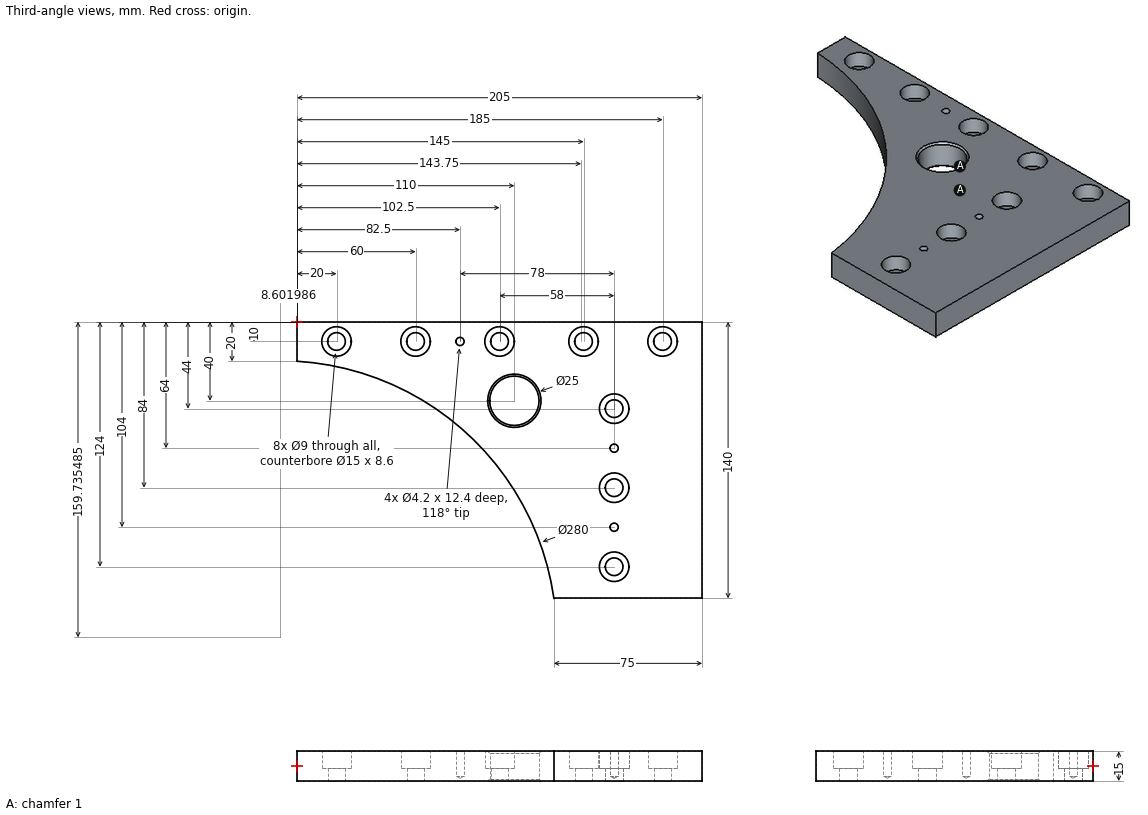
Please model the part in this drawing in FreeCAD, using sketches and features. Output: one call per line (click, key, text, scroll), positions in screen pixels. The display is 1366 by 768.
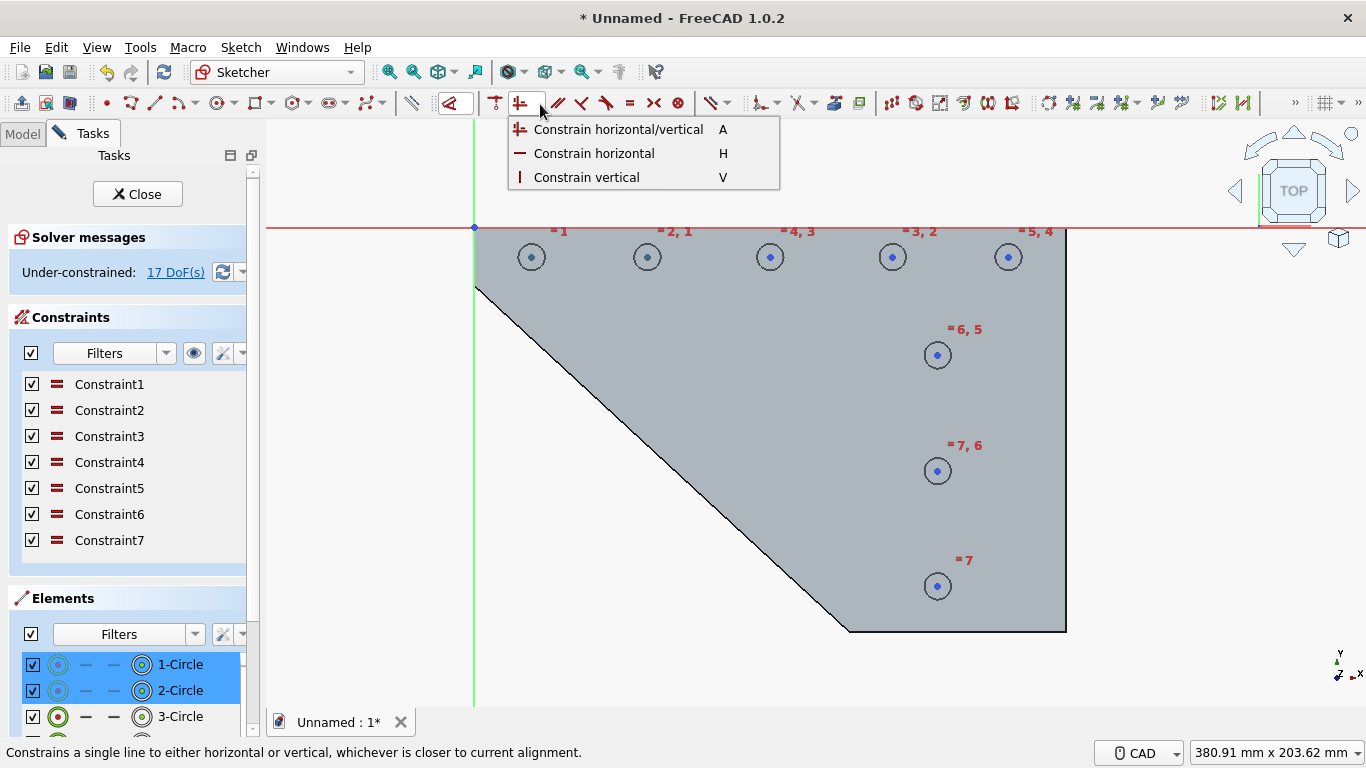
click(644, 153)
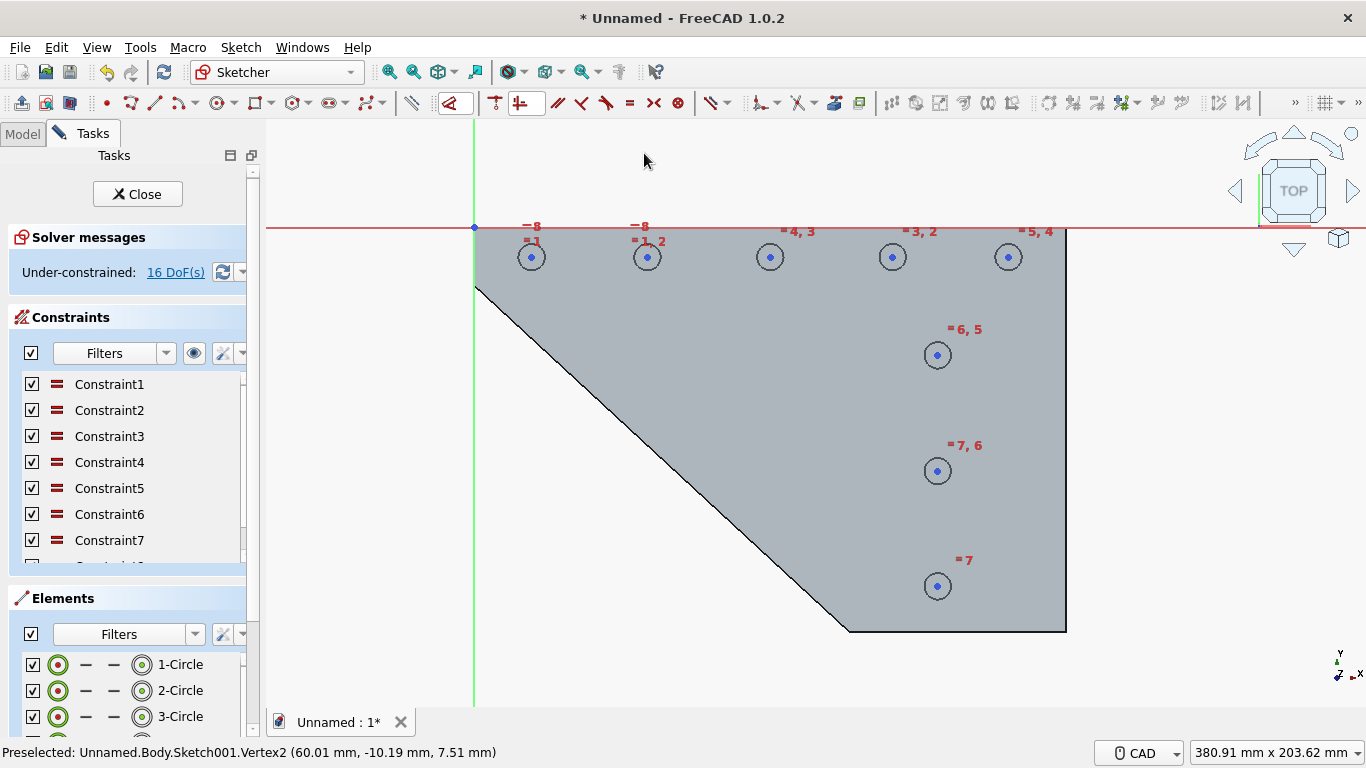
click(647, 257)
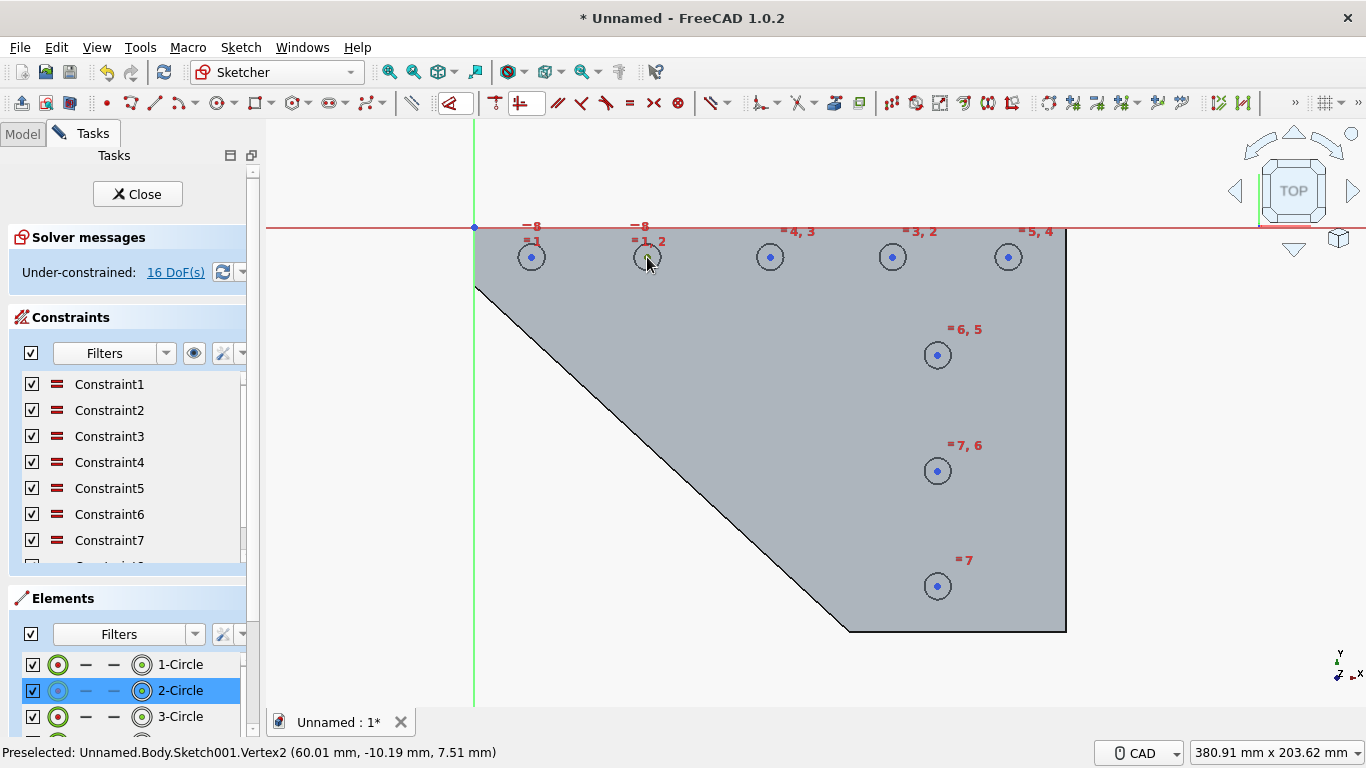
click(893, 257)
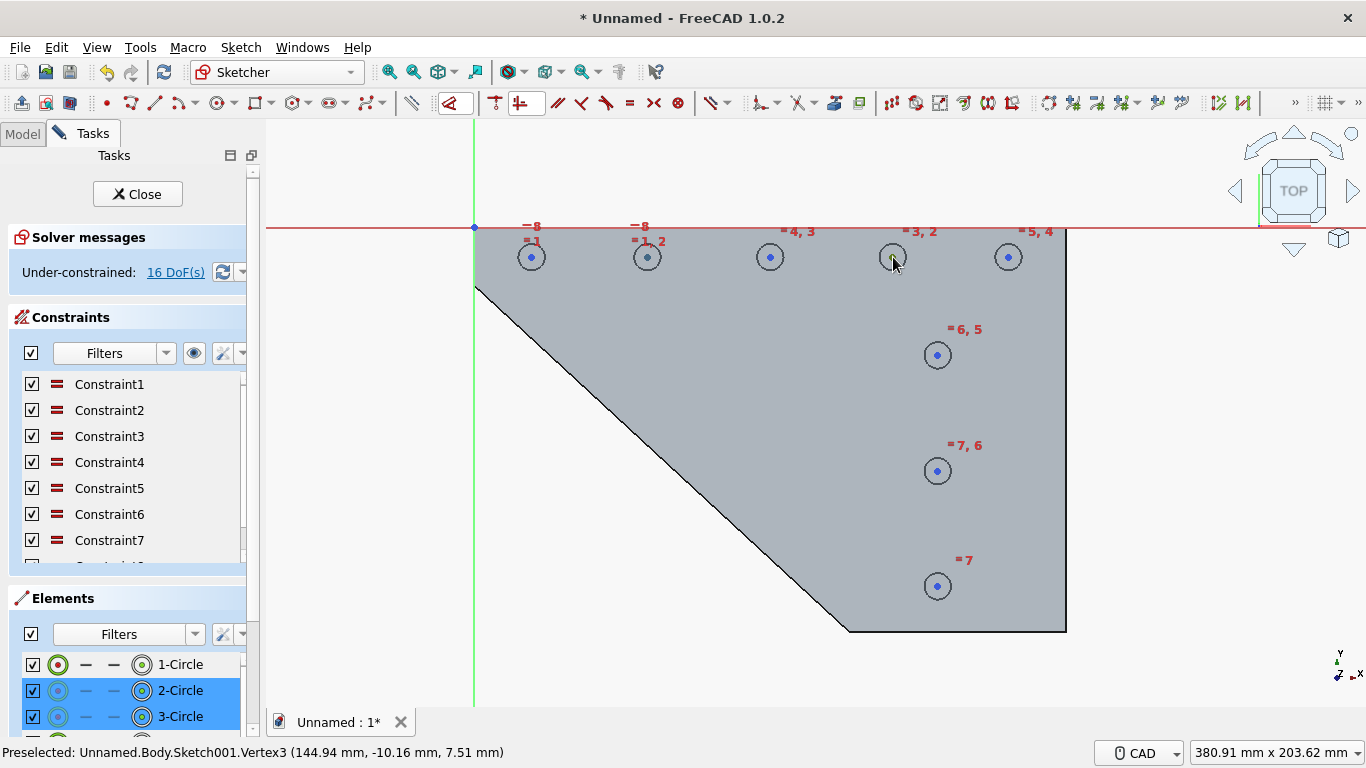
click(540, 104)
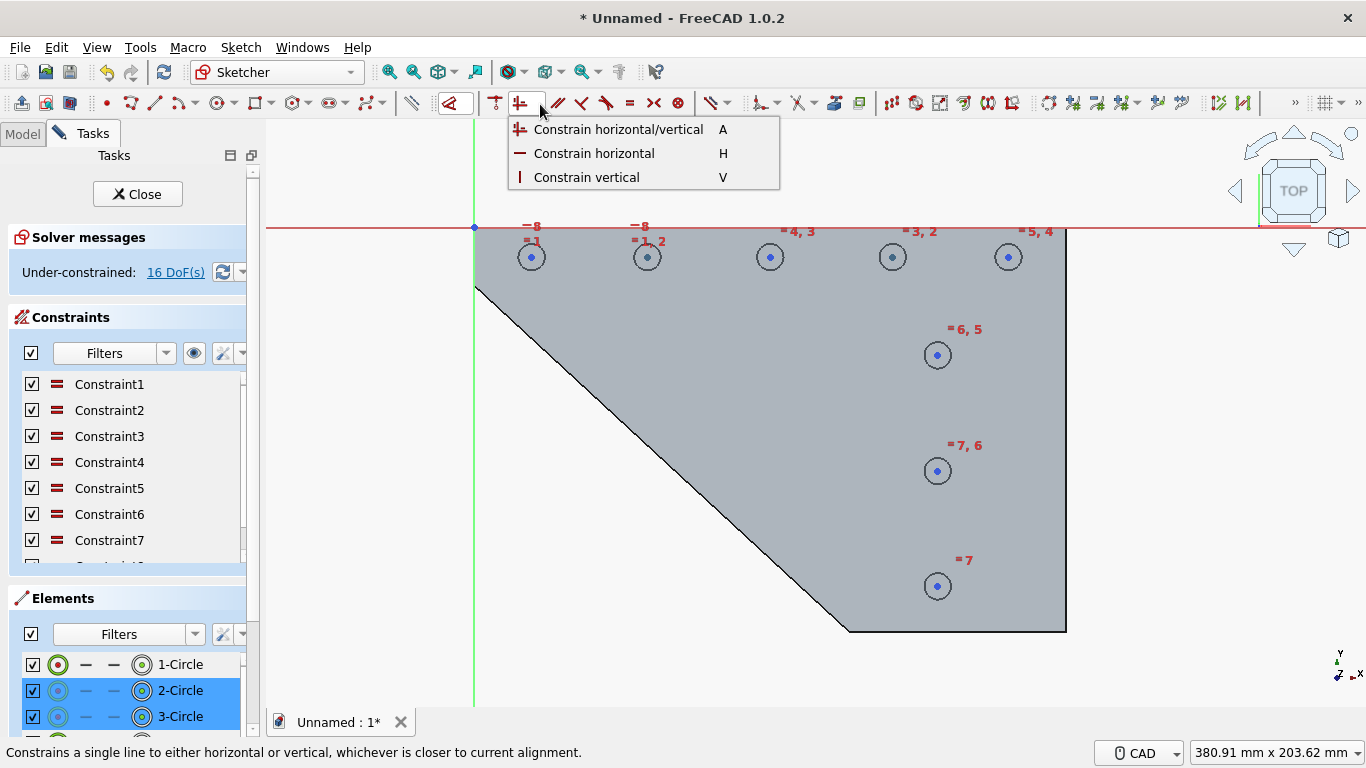
click(644, 153)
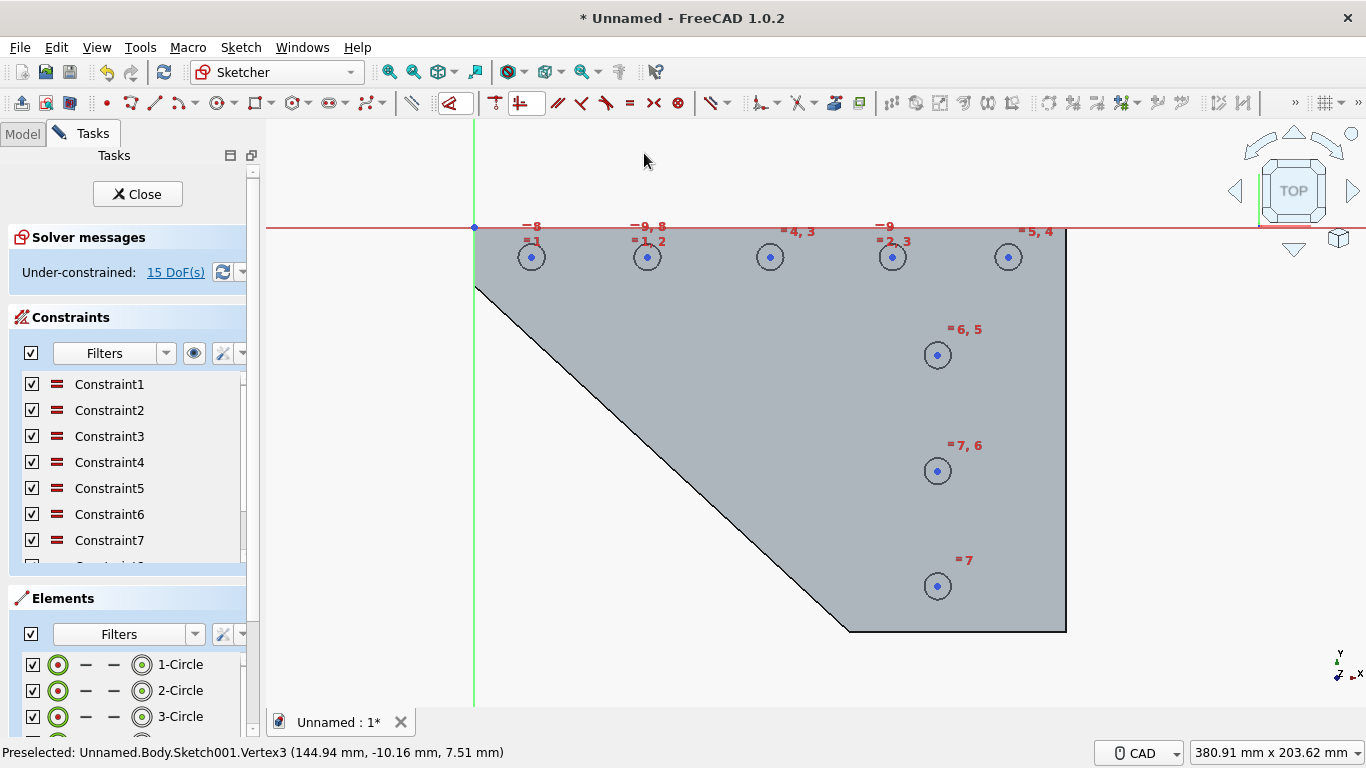
click(647, 257)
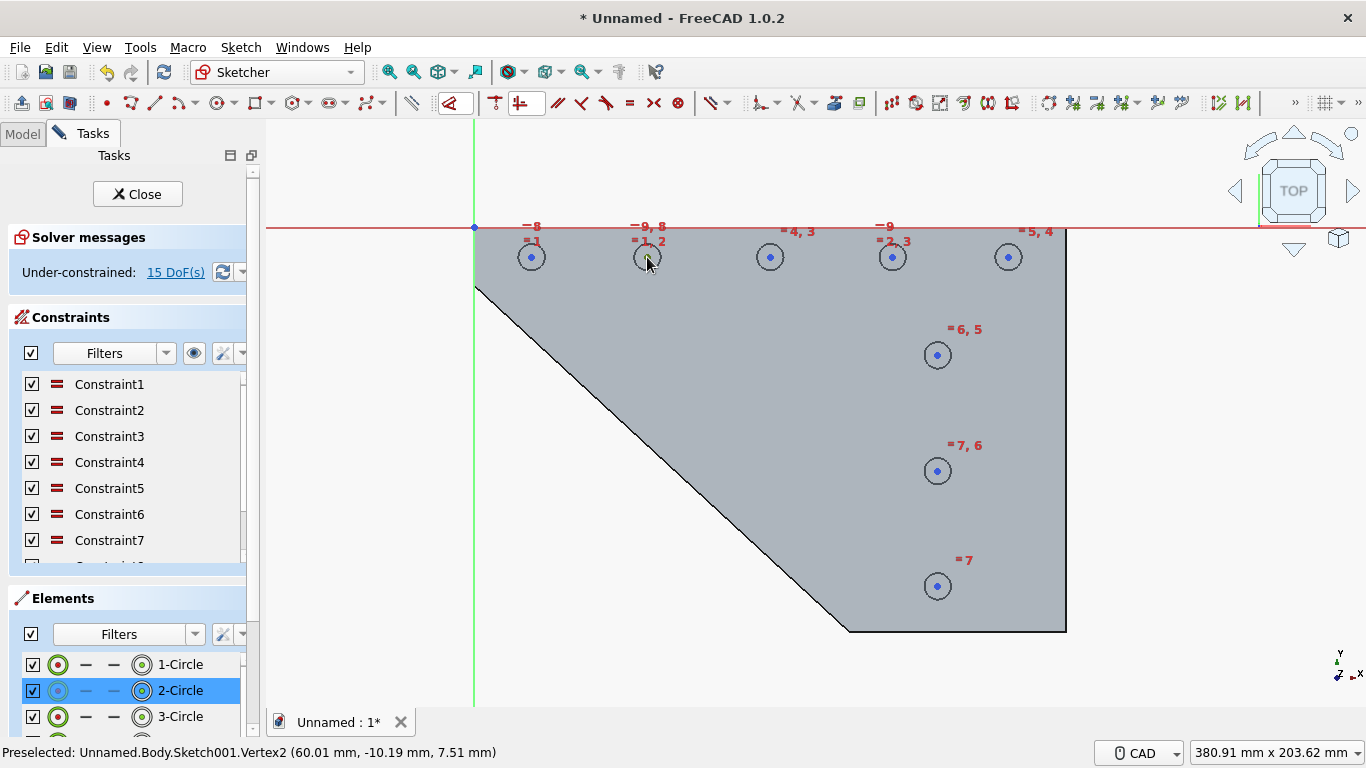
click(770, 257)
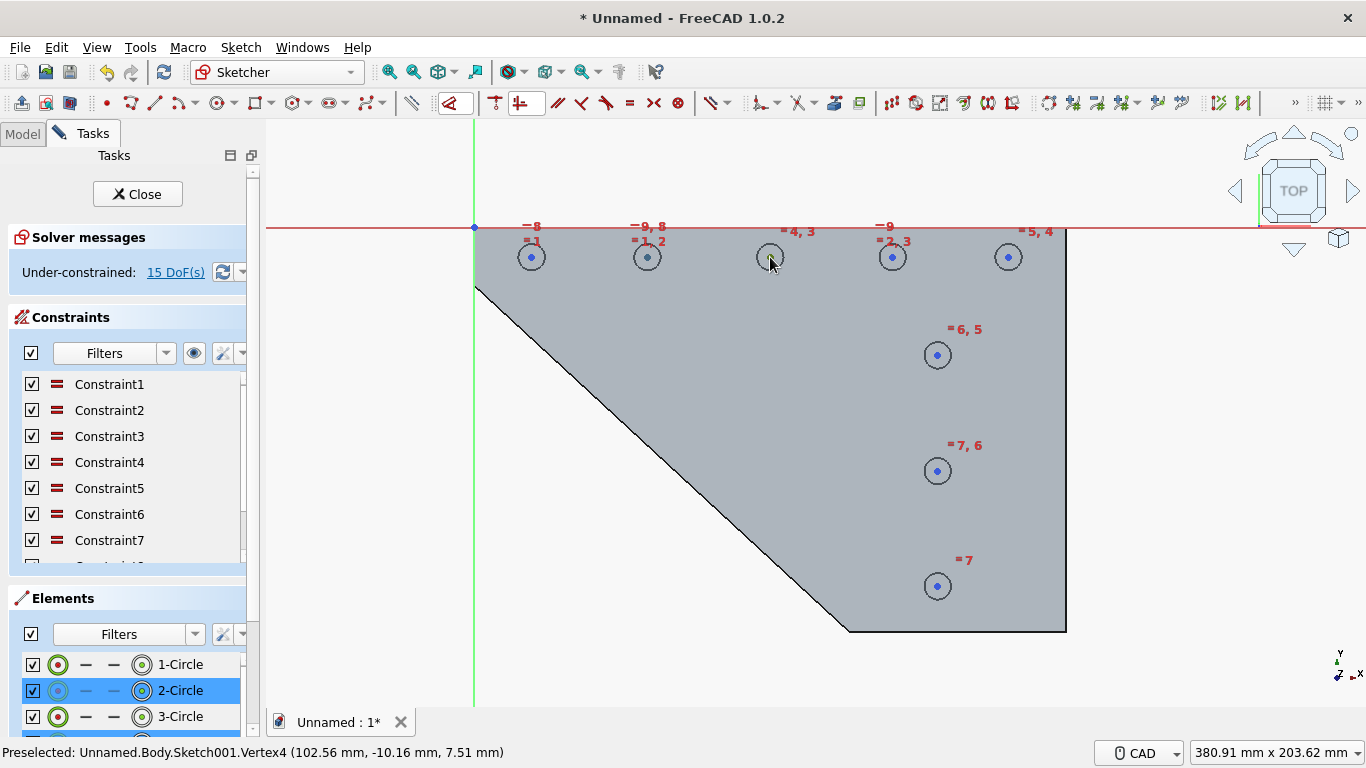
click(540, 104)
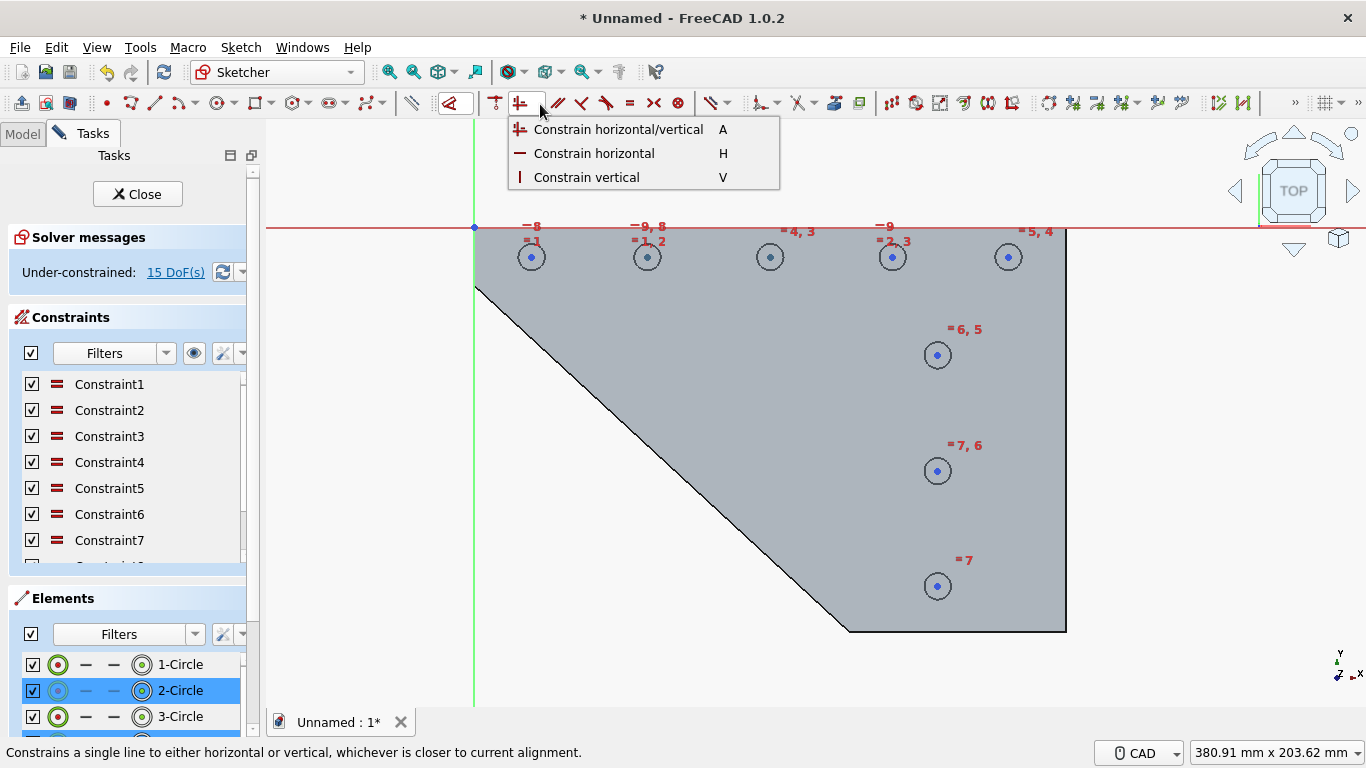
click(644, 153)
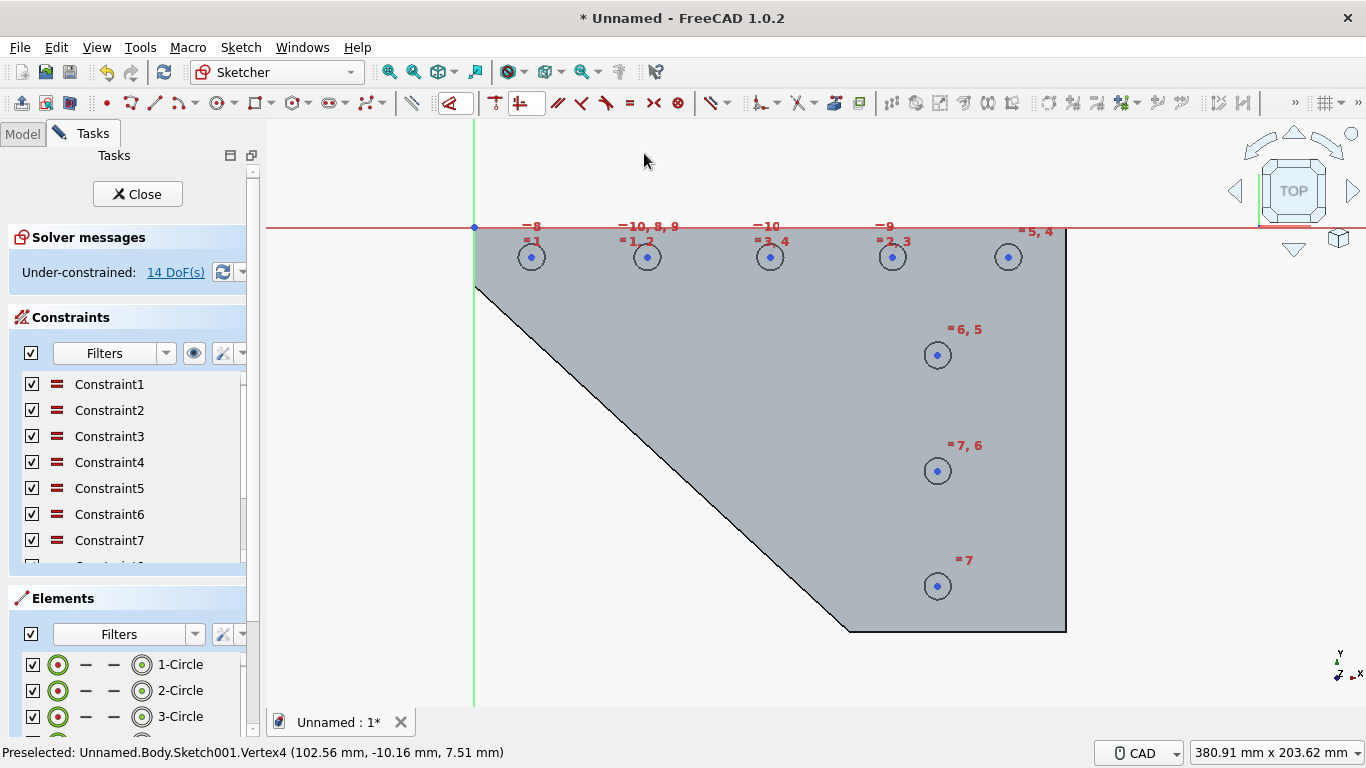
click(893, 257)